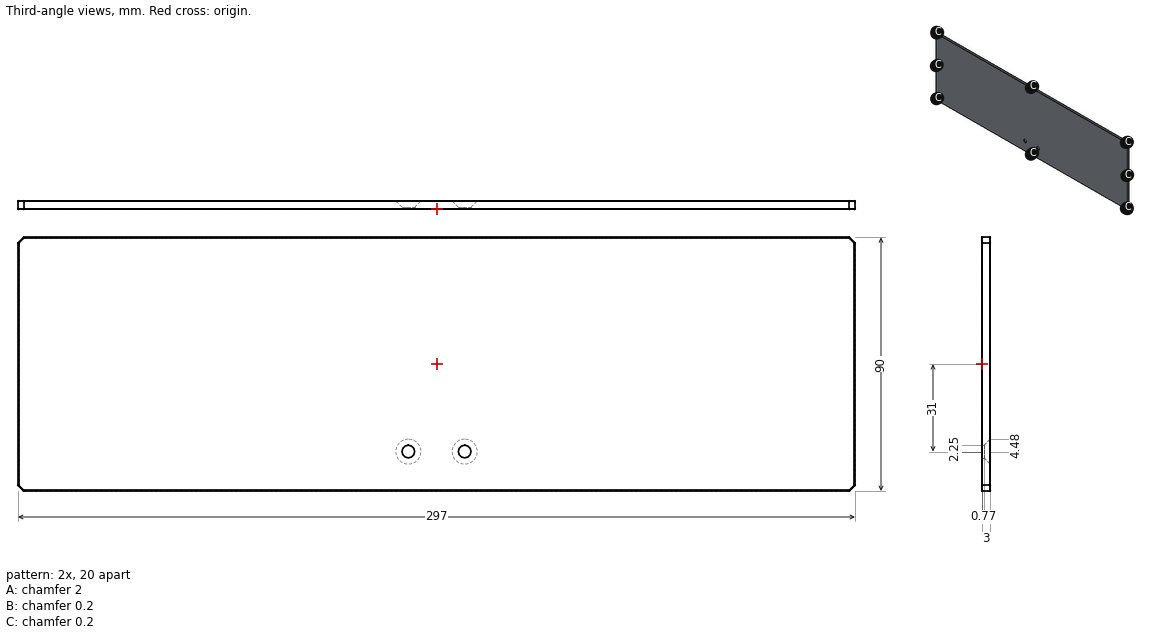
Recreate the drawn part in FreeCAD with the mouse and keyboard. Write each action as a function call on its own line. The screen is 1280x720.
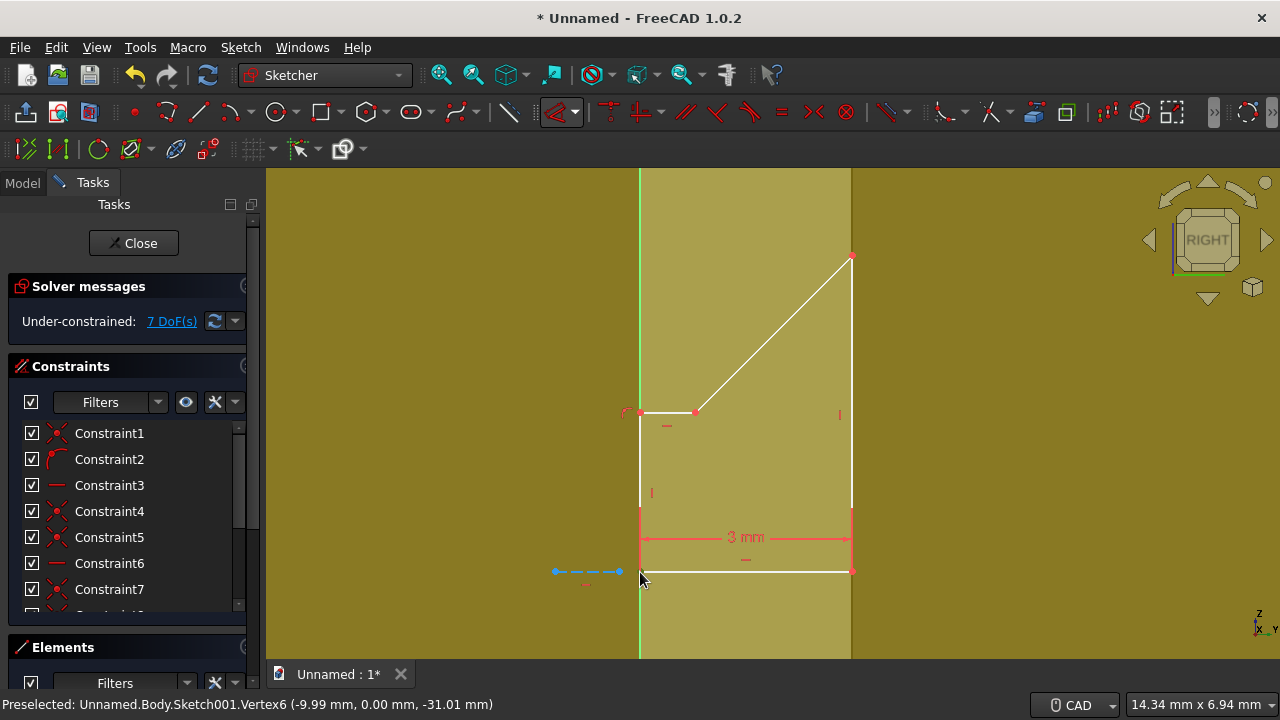
key(i)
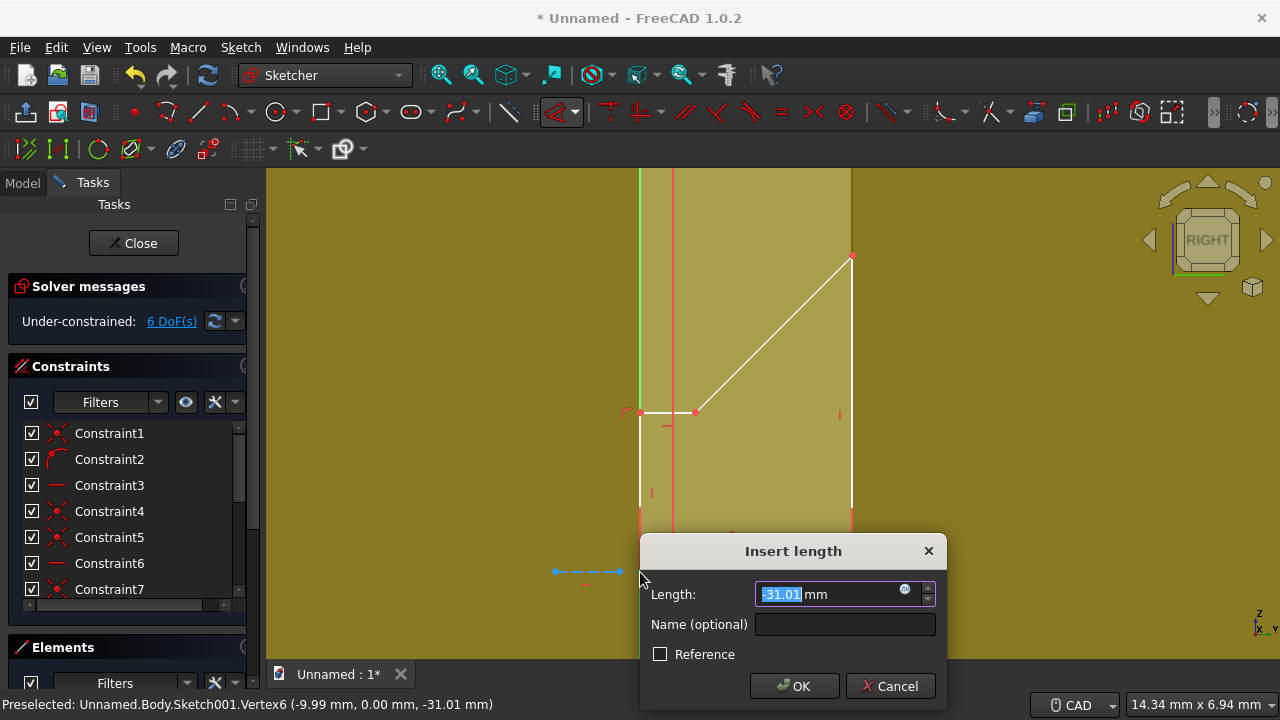
text(-31)
key(Return)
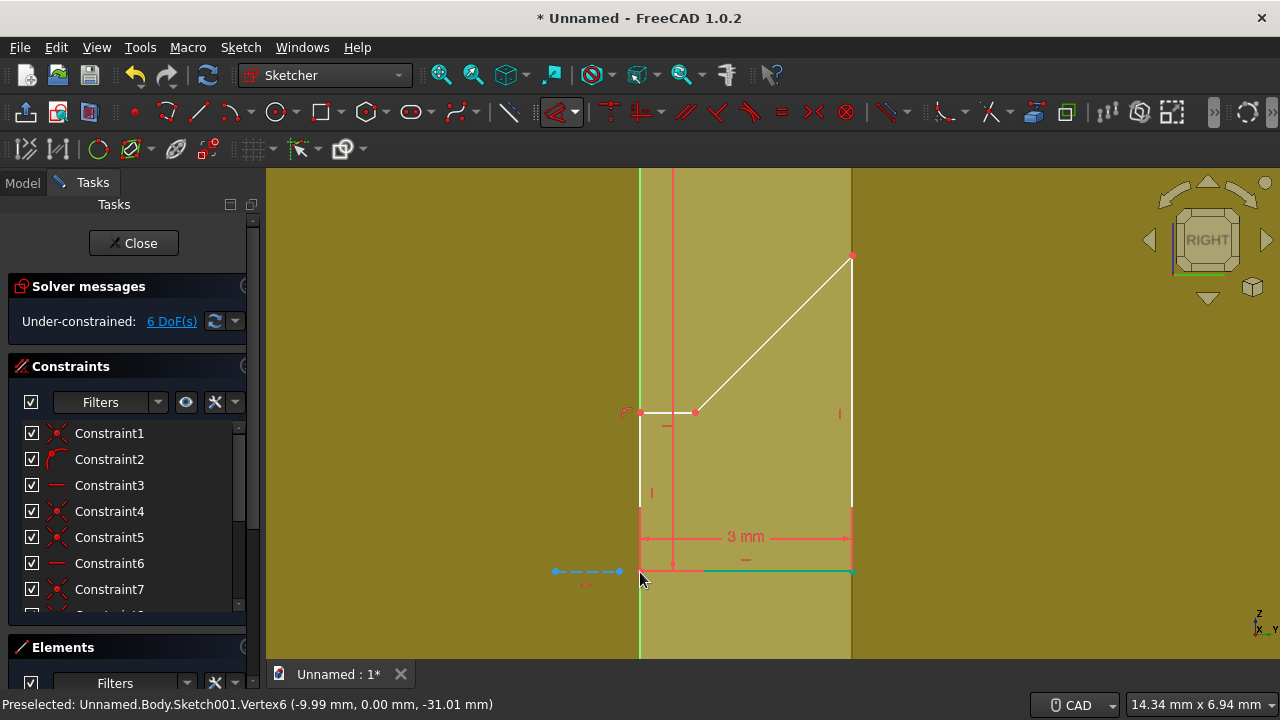
click(619, 572)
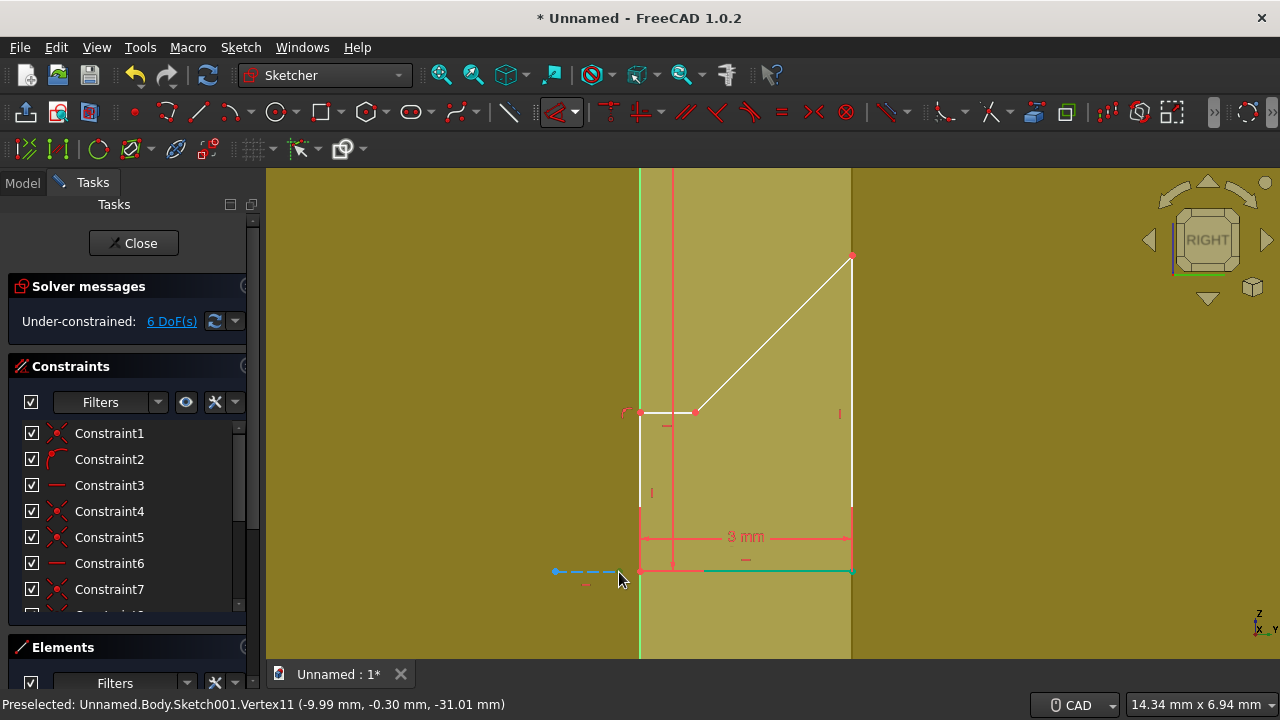
key(i)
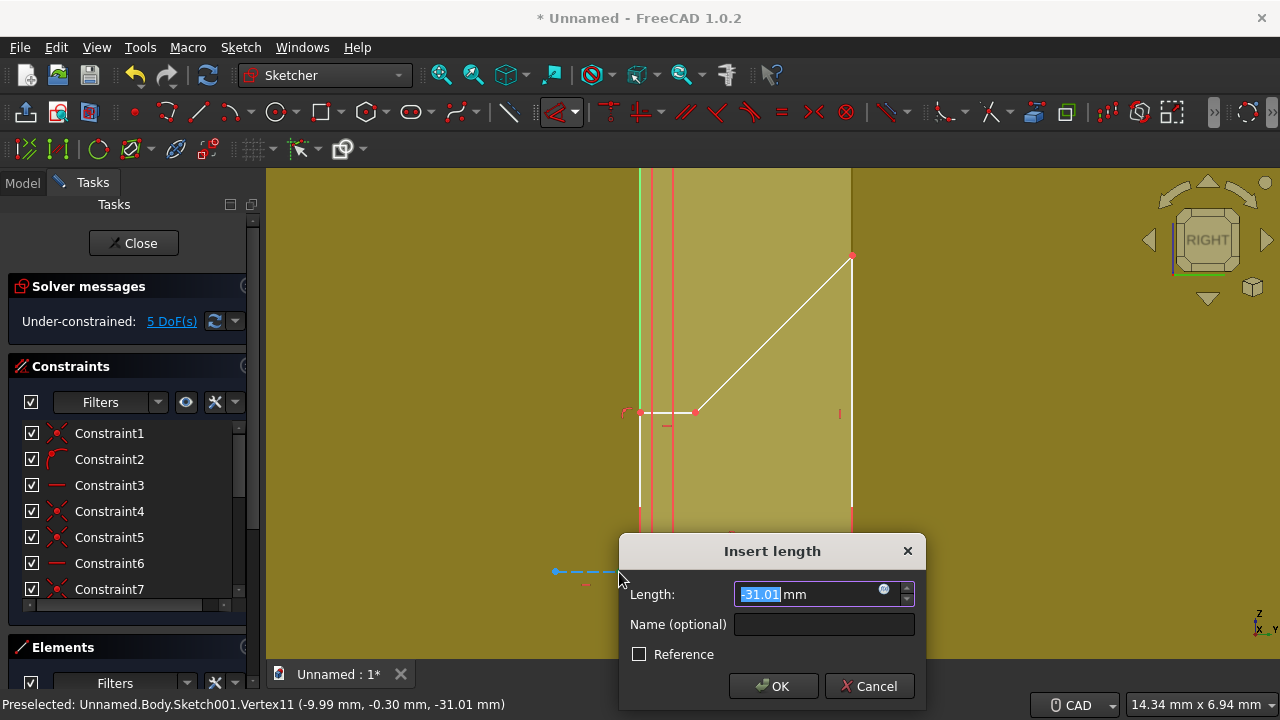
text(-31)
key(Return)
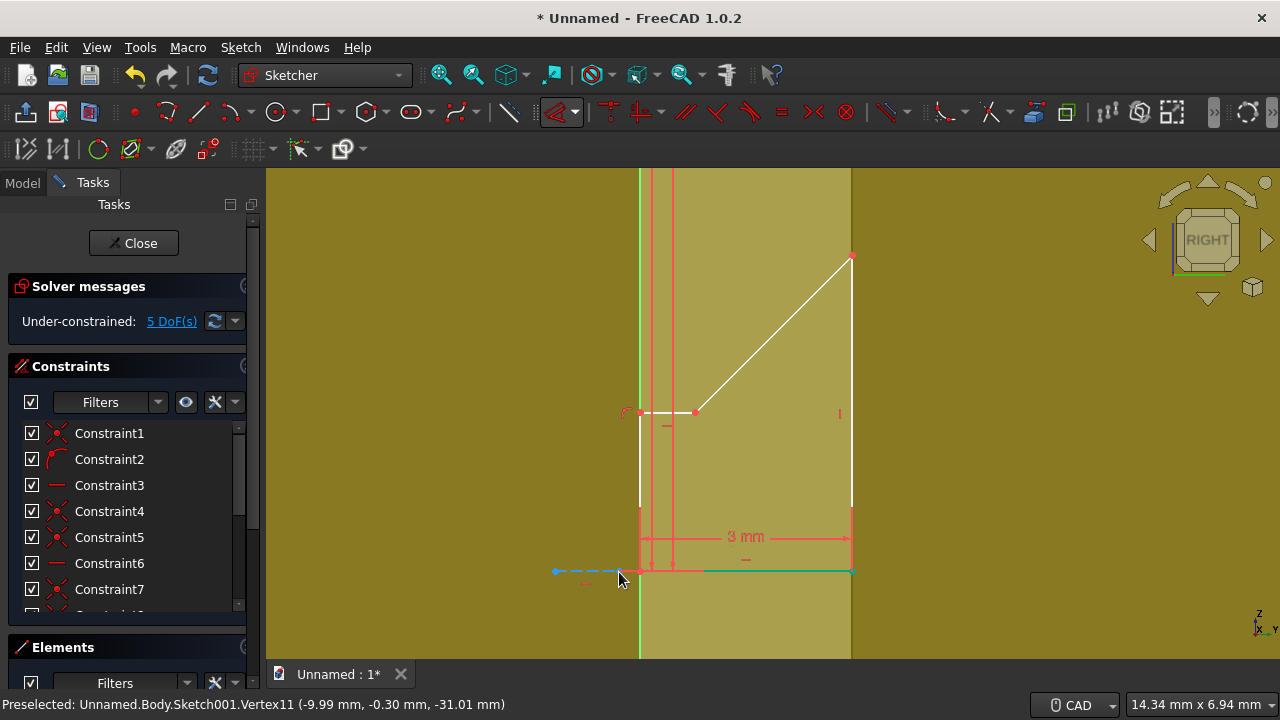
click(679, 413)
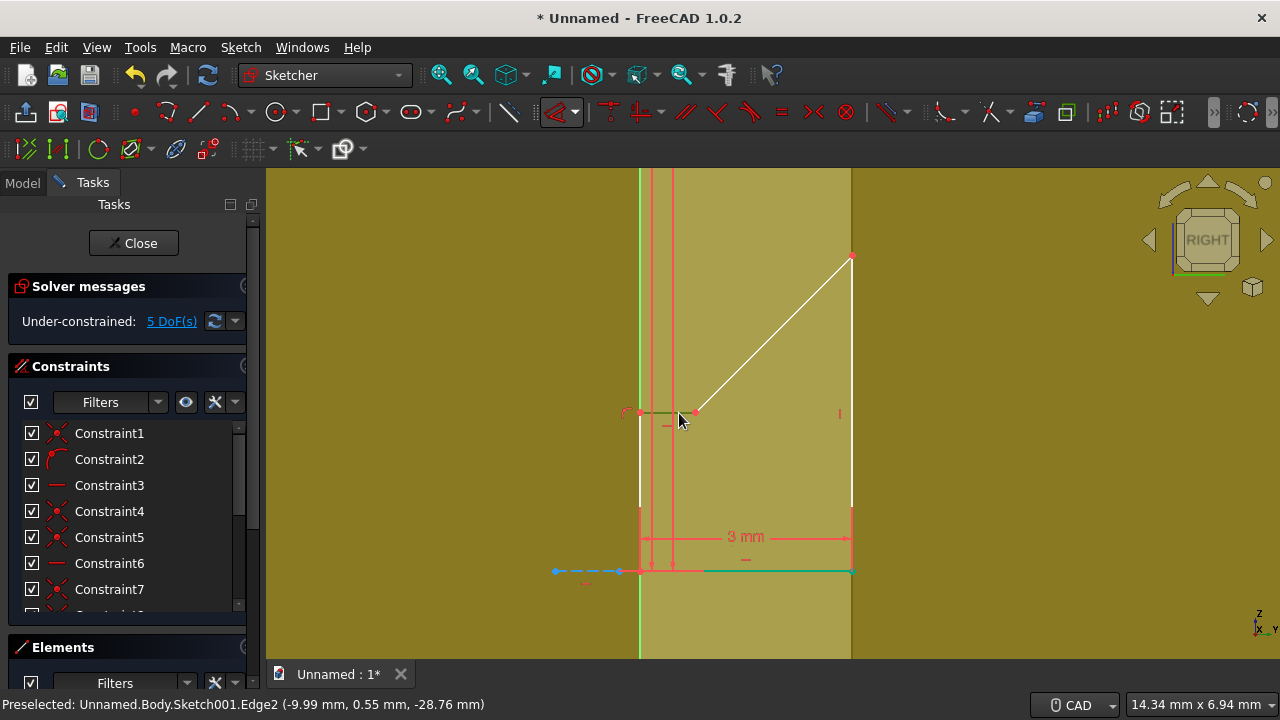
key(l)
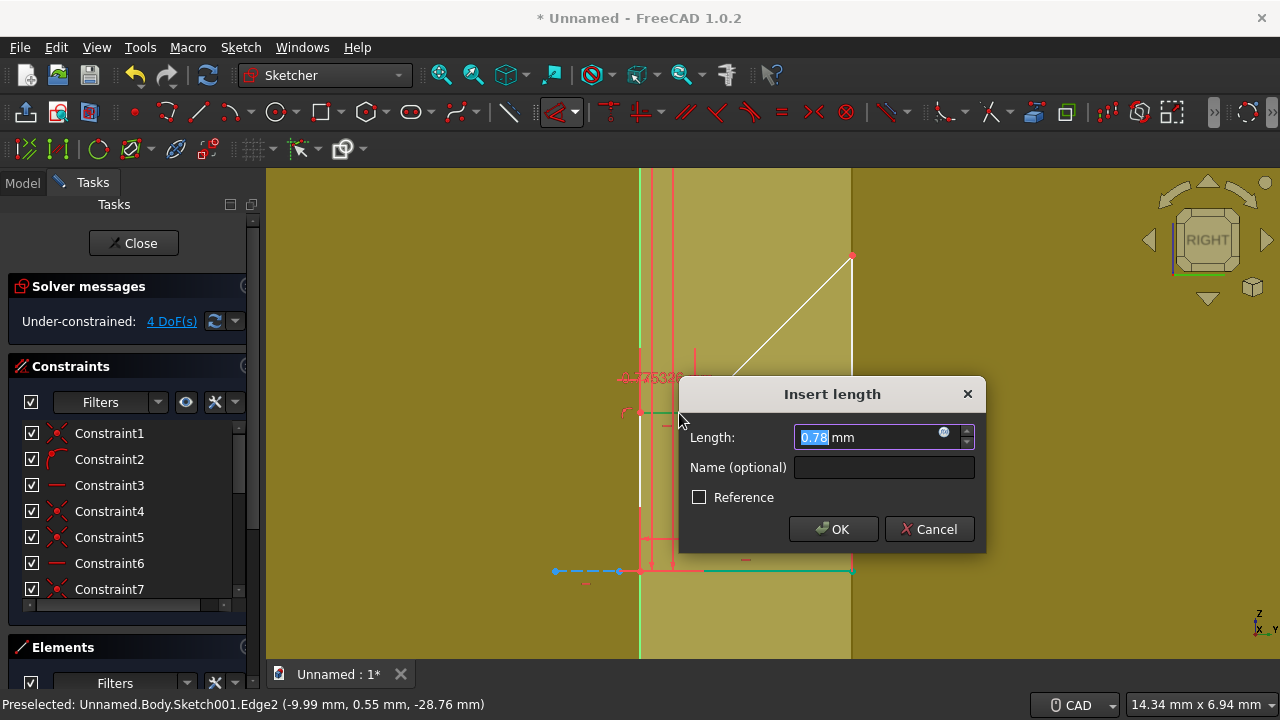
text(0.77)
key(Return)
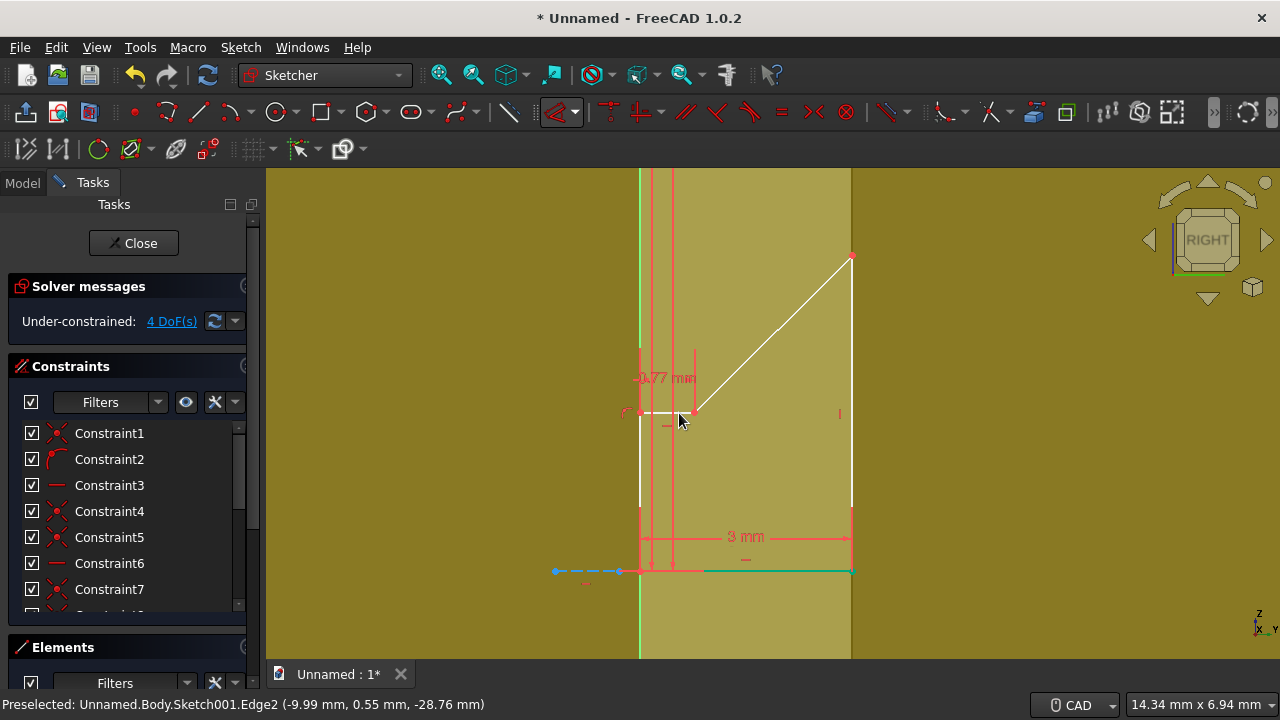
click(640, 461)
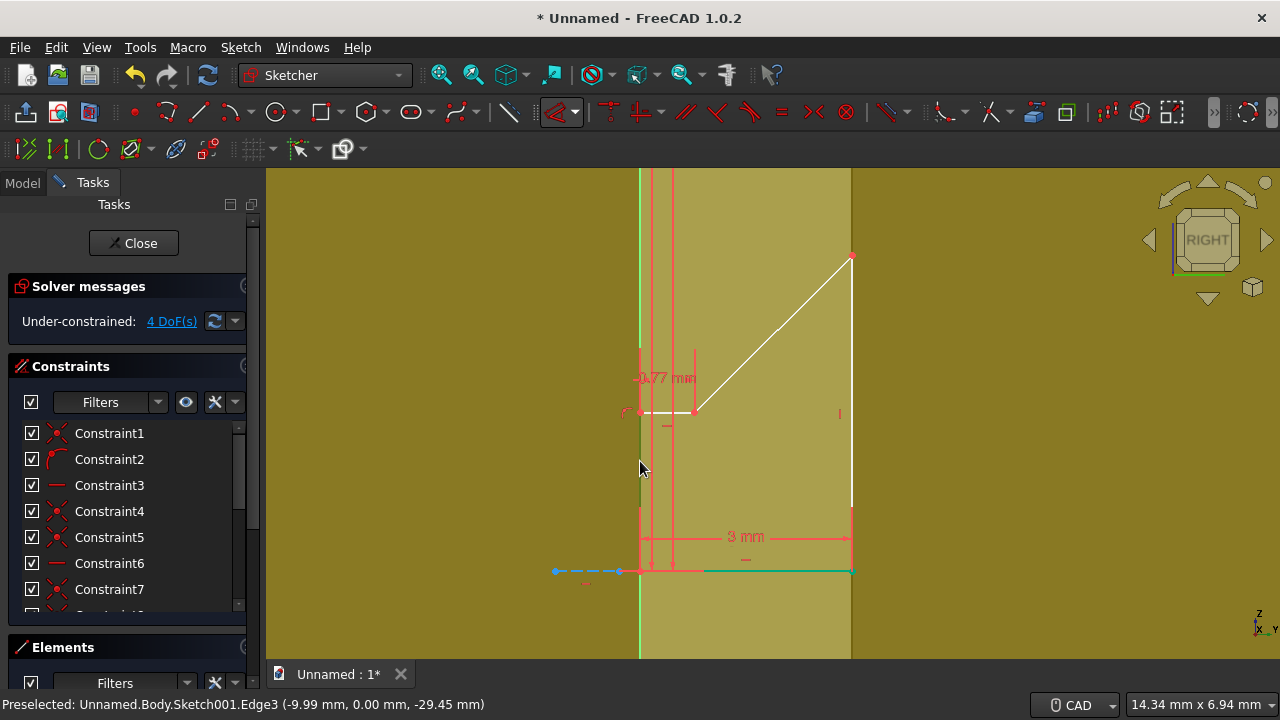
key(i)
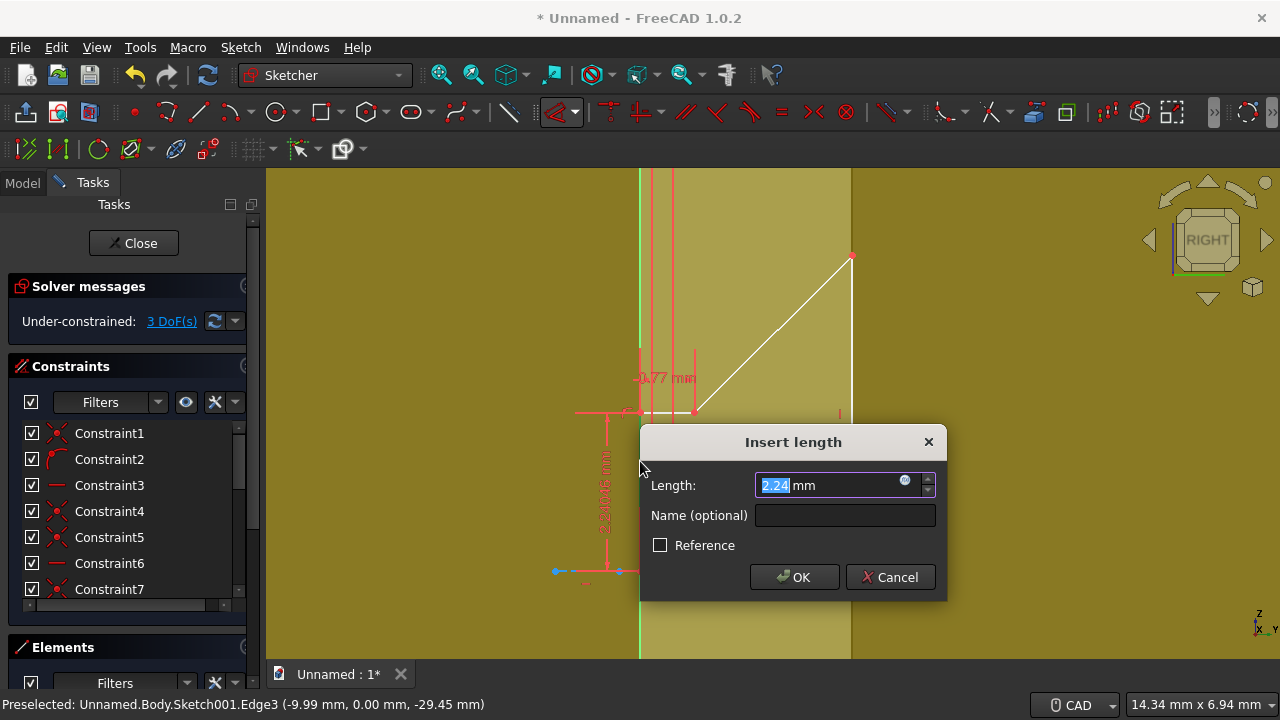
text(2.25)
key(Return)